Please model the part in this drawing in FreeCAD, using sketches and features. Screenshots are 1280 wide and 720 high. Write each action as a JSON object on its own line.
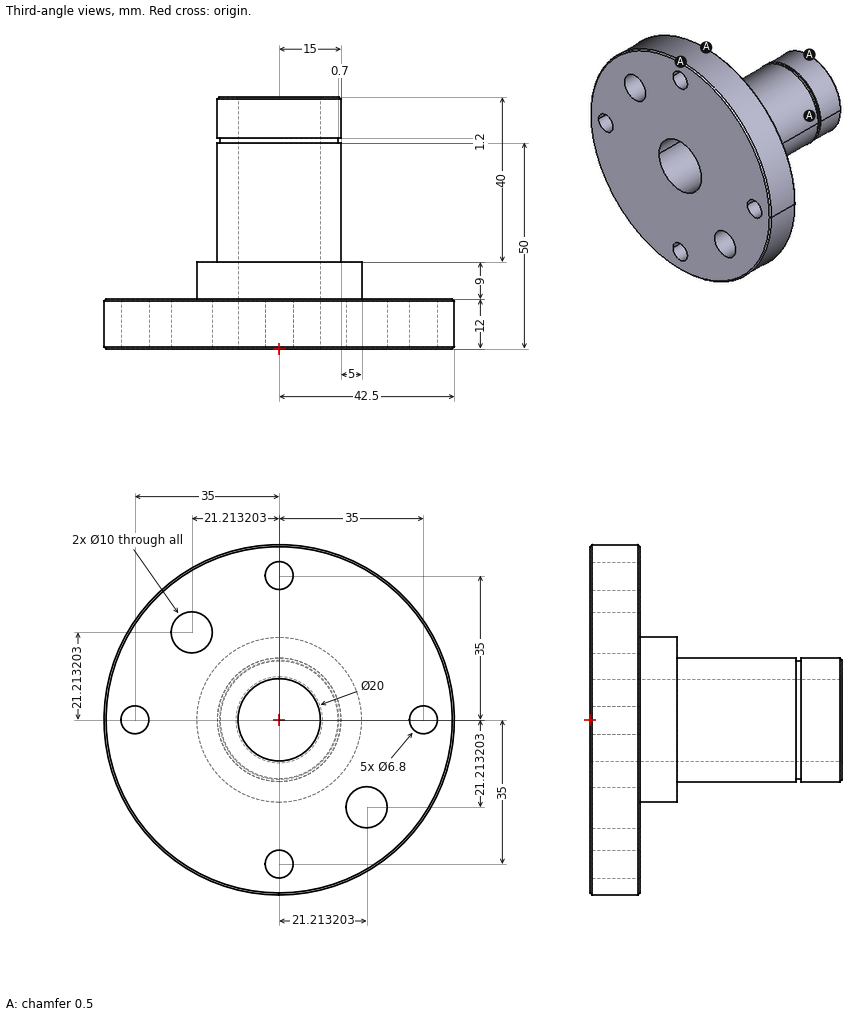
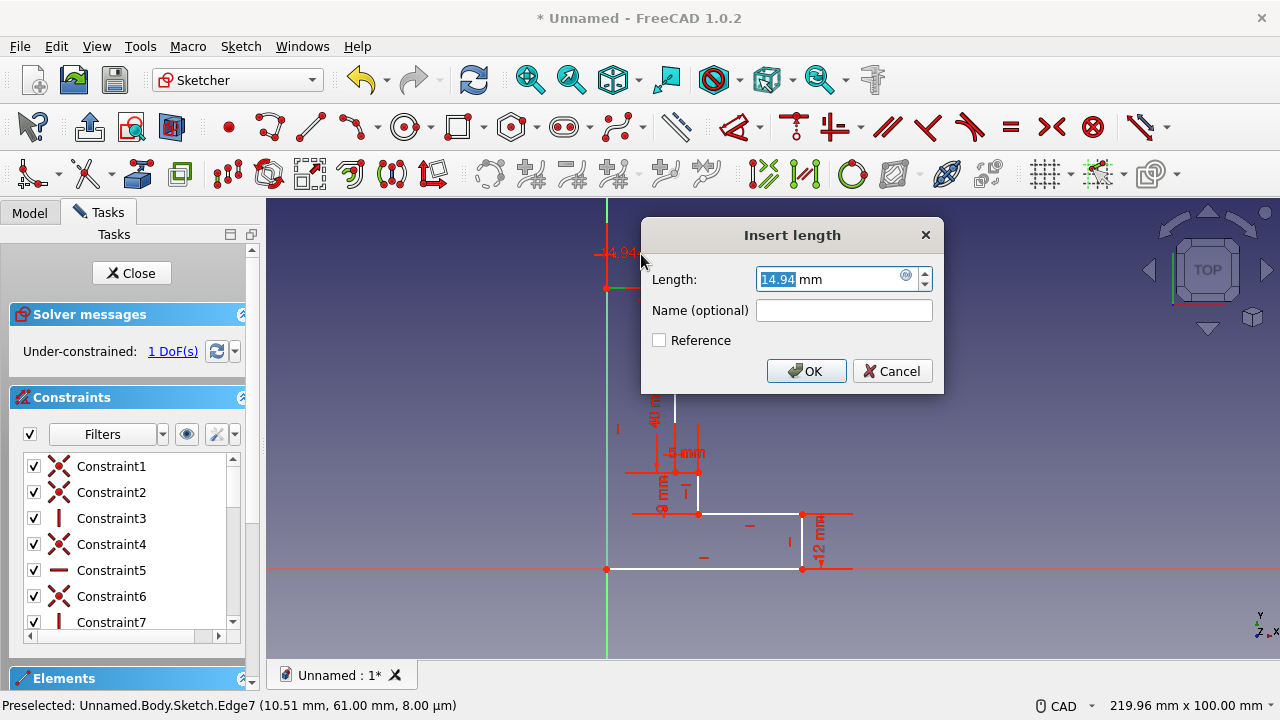
{"action": "type", "text": "15"}
{"action": "key", "text": "Return"}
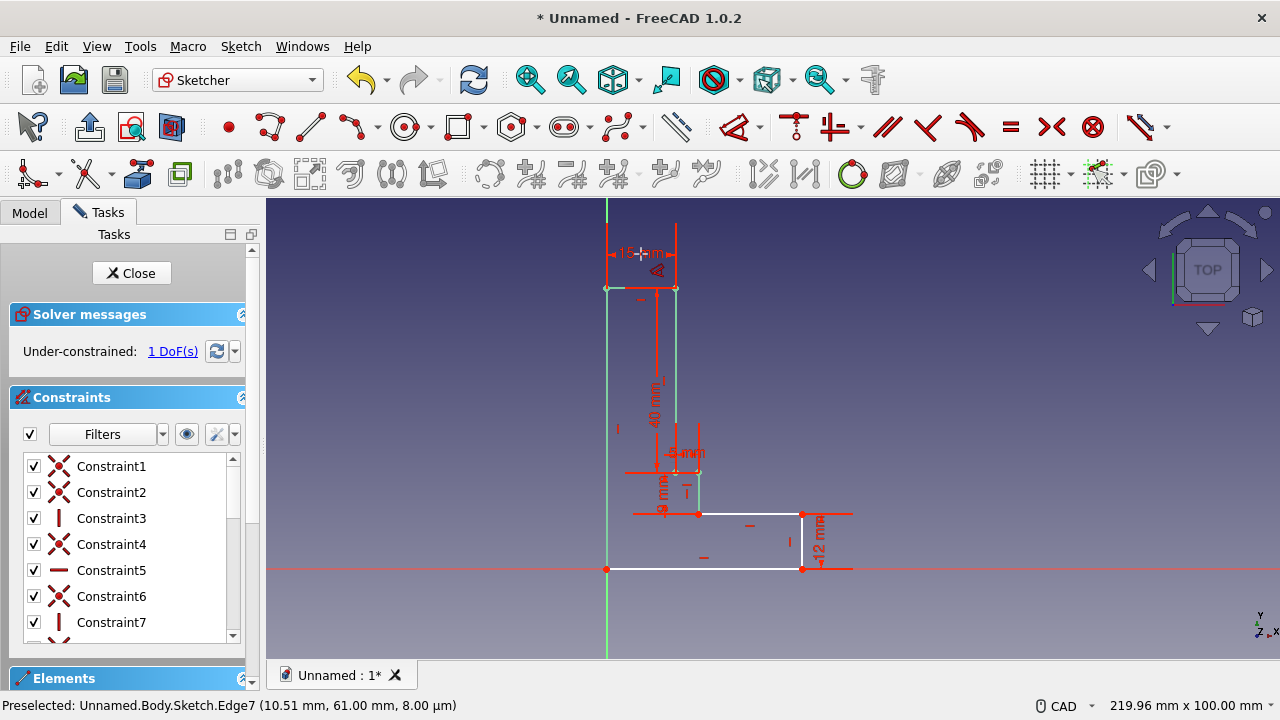
{"action": "left_click", "coordinate": [665, 569]}
{"action": "left_click", "coordinate": [705, 603]}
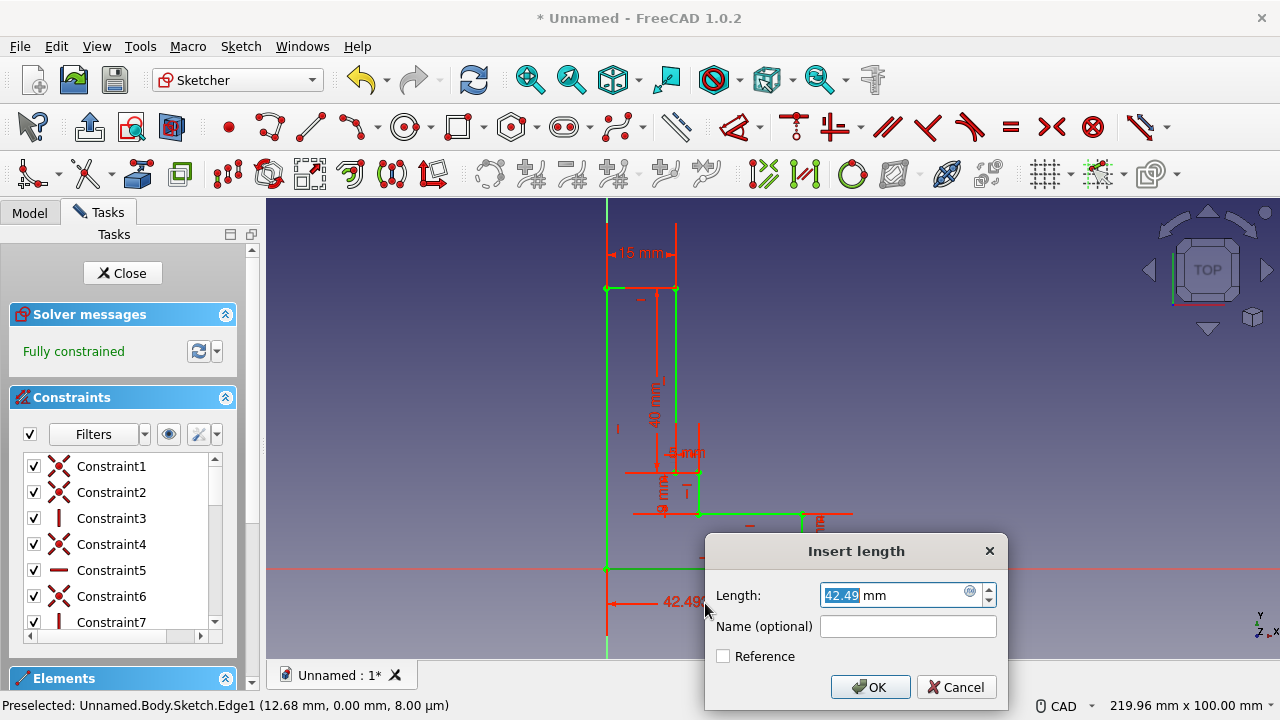
{"action": "type", "text": "42.5"}
{"action": "key", "text": "Return"}
{"action": "key", "text": "Escape"}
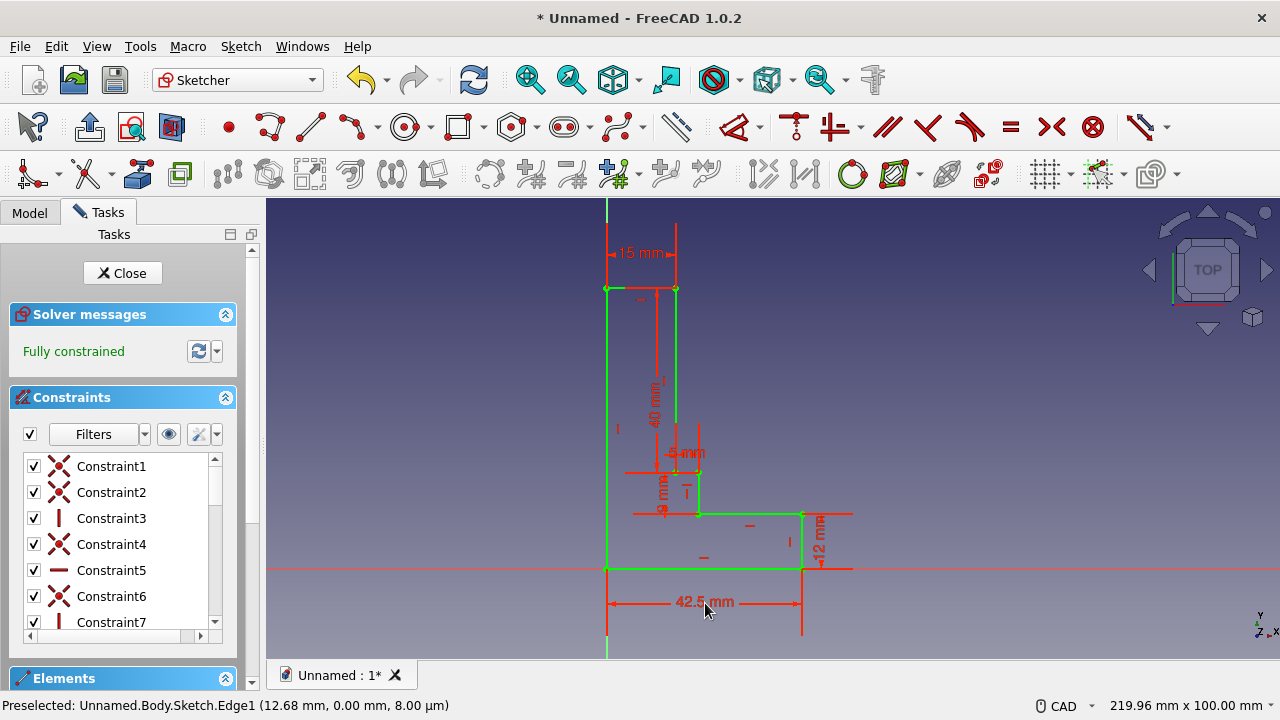
{"action": "left_click", "coordinate": [123, 273]}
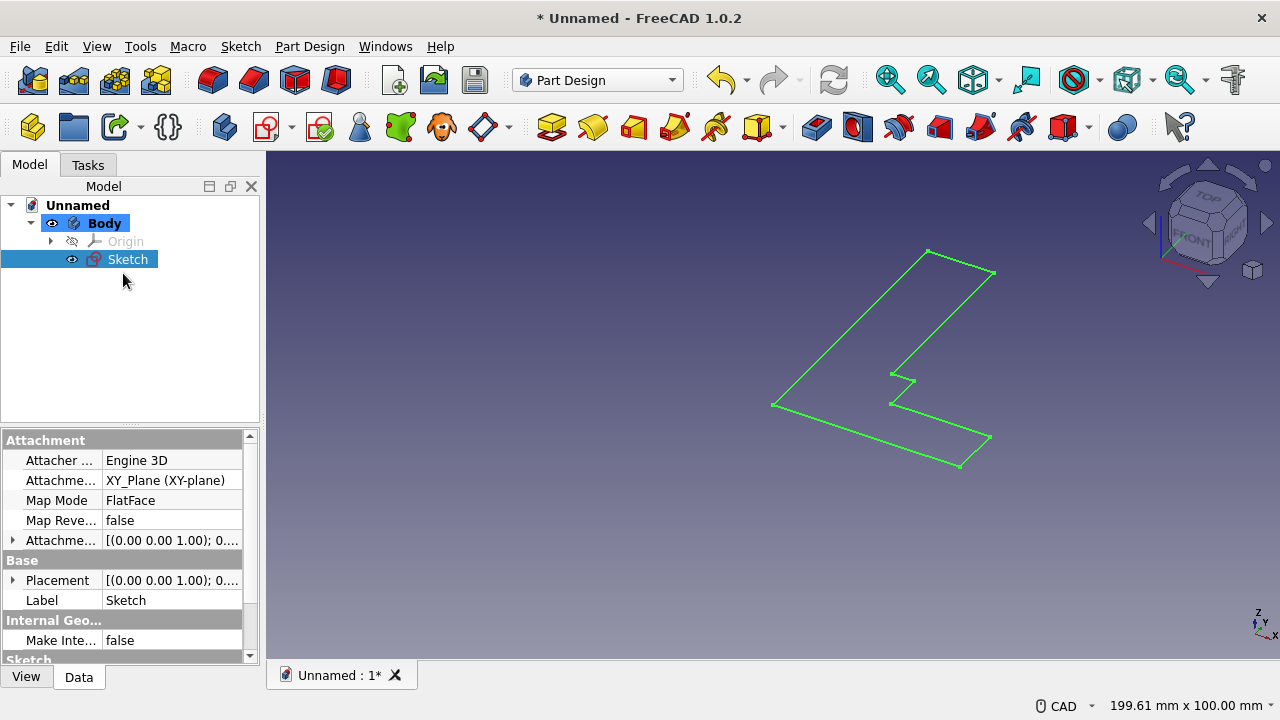
{"action": "left_click", "coordinate": [593, 128]}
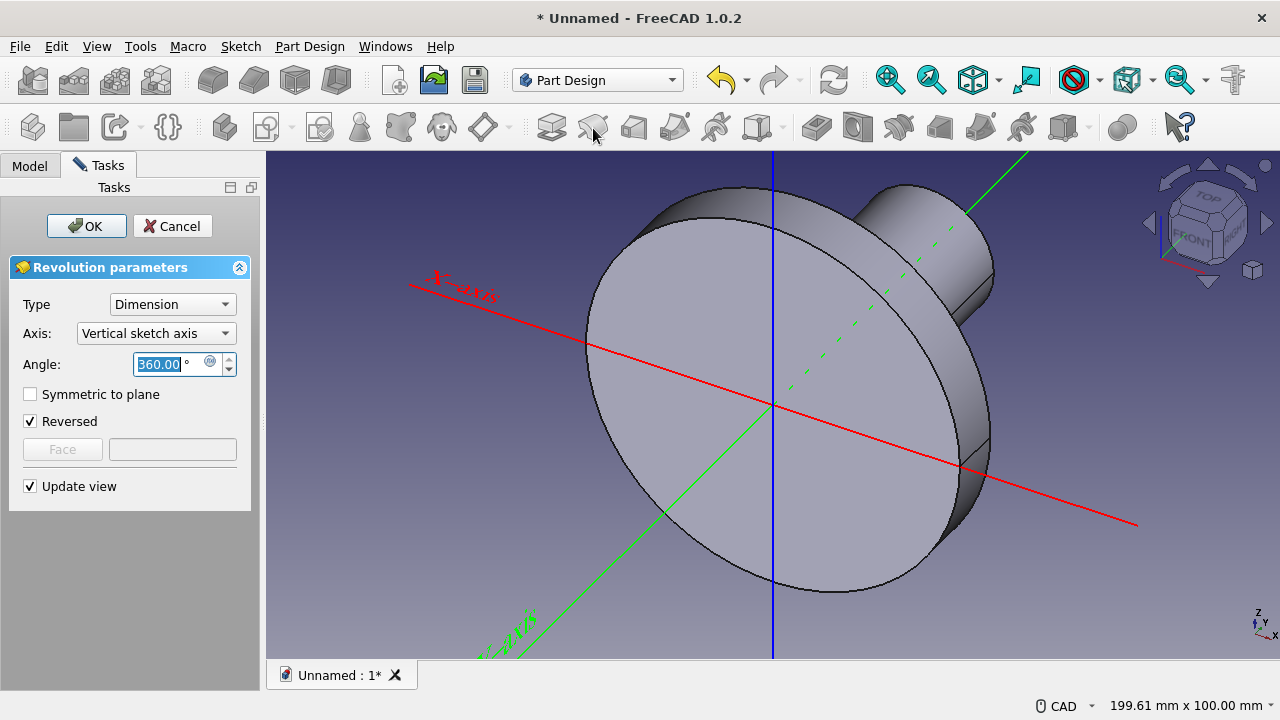
{"action": "left_click", "coordinate": [87, 226]}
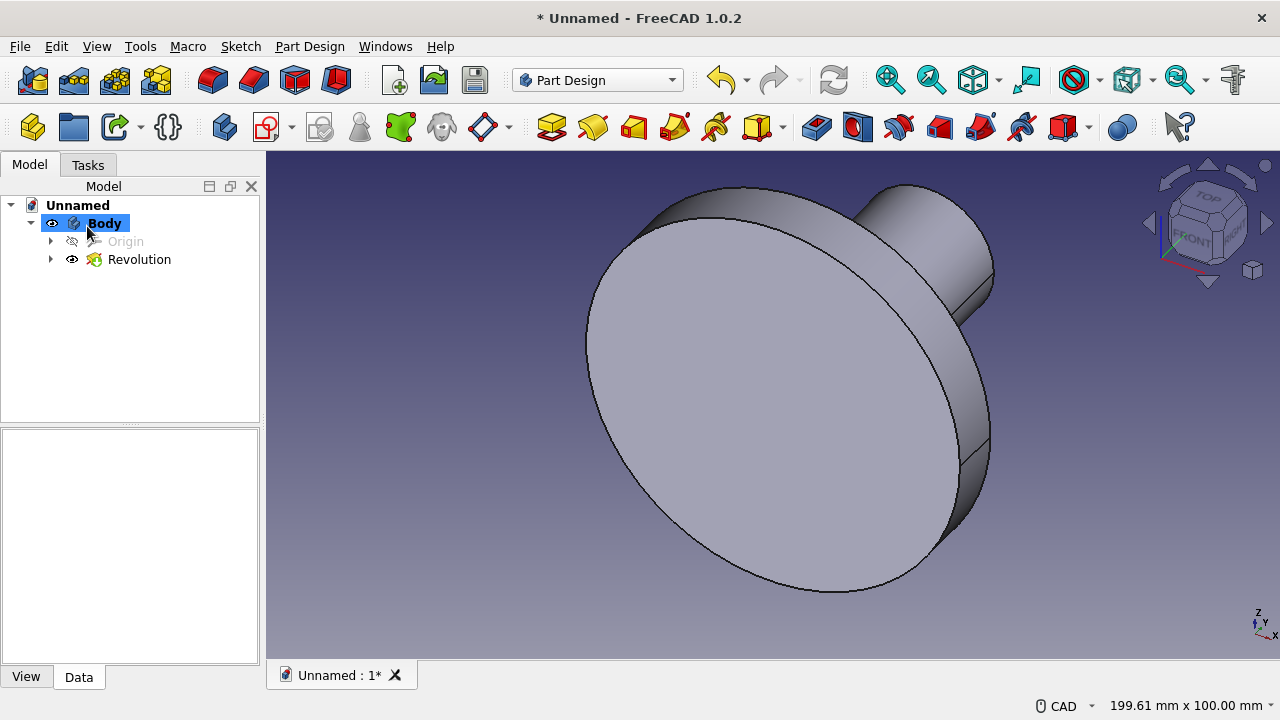
{"action": "key", "text": "v f"}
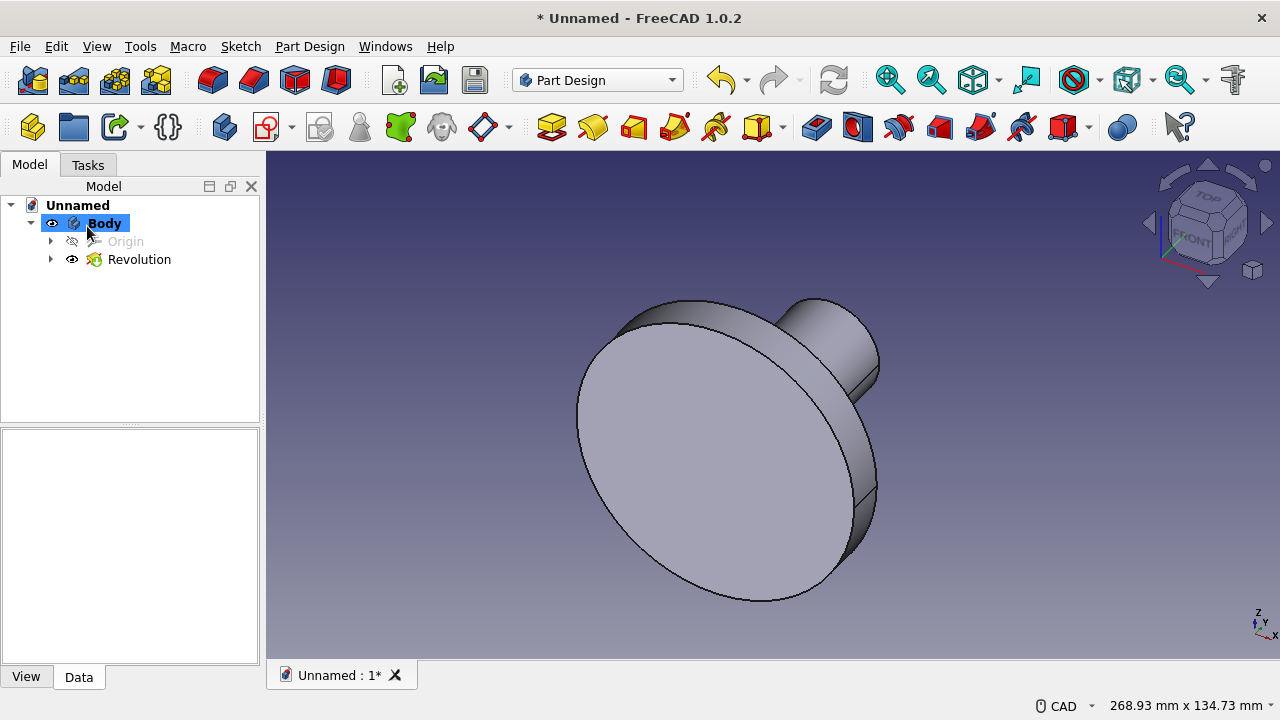
{"action": "key", "text": "4"}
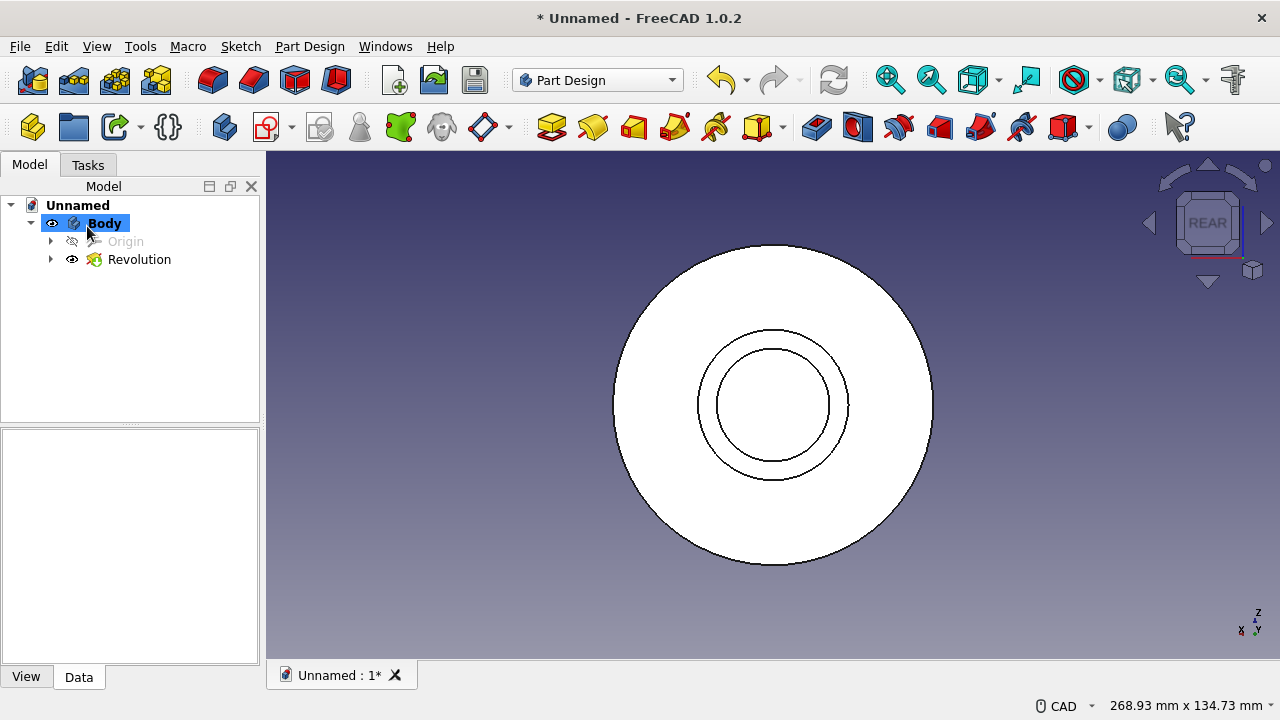
{"action": "left_click", "coordinate": [773, 404]}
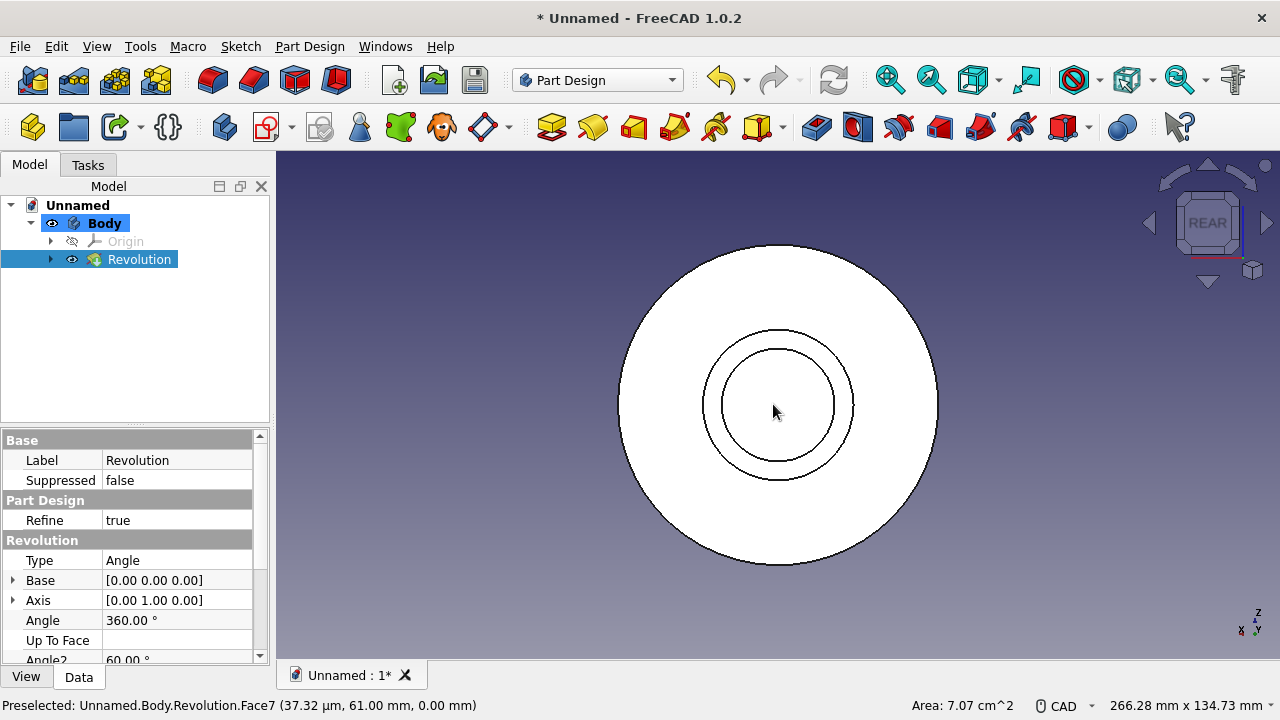
{"action": "left_click", "coordinate": [266, 128]}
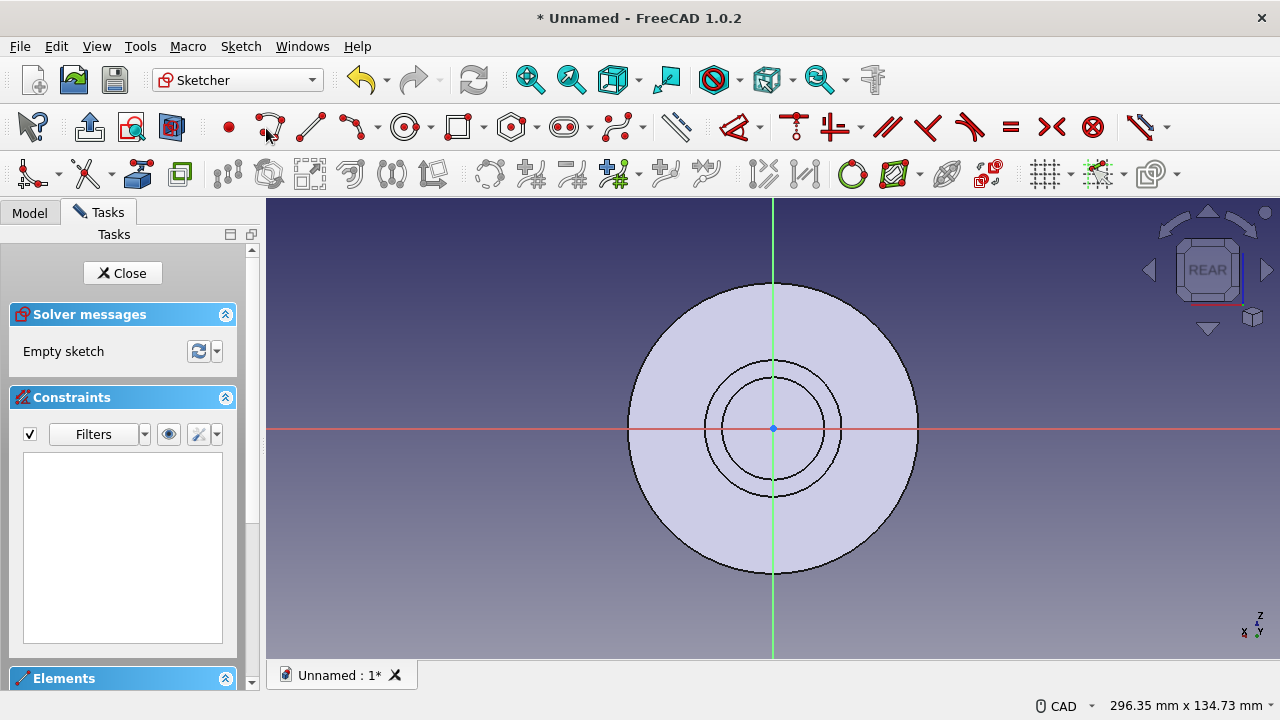
{"action": "scroll", "coordinate": [796, 428], "scroll_direction": "up", "scroll_amount": 7}